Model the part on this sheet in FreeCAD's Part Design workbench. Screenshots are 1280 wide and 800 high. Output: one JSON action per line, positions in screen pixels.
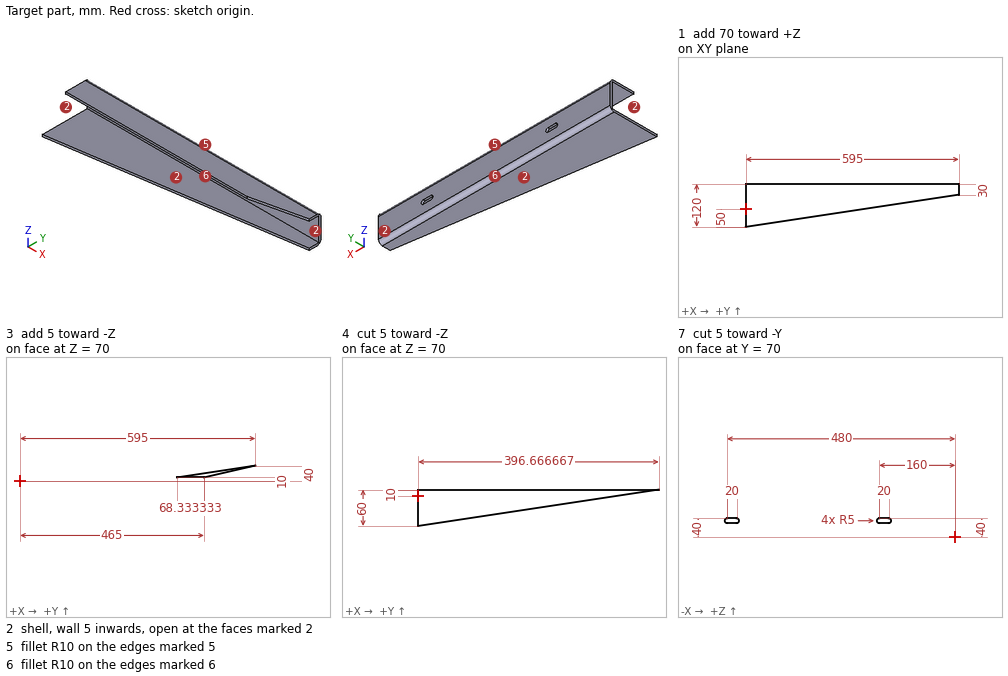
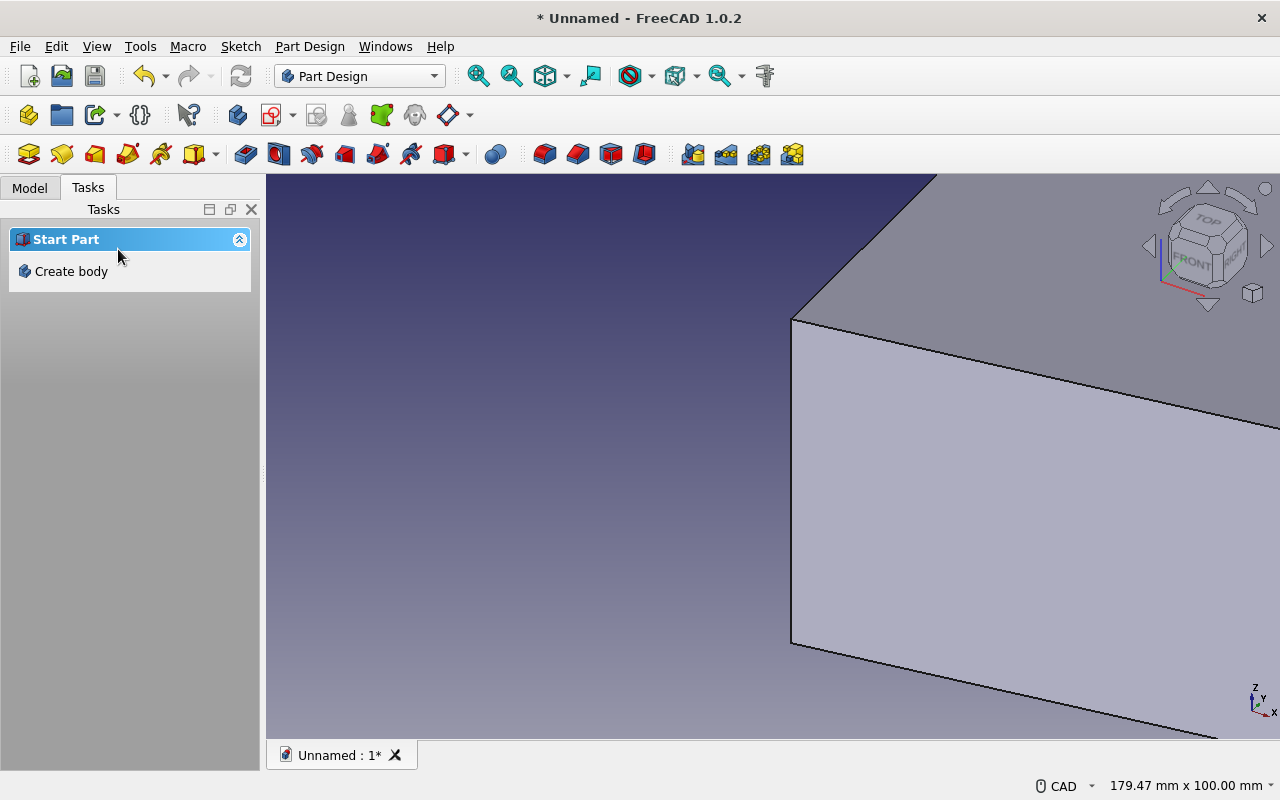
{"action": "left_click", "coordinate": [479, 76]}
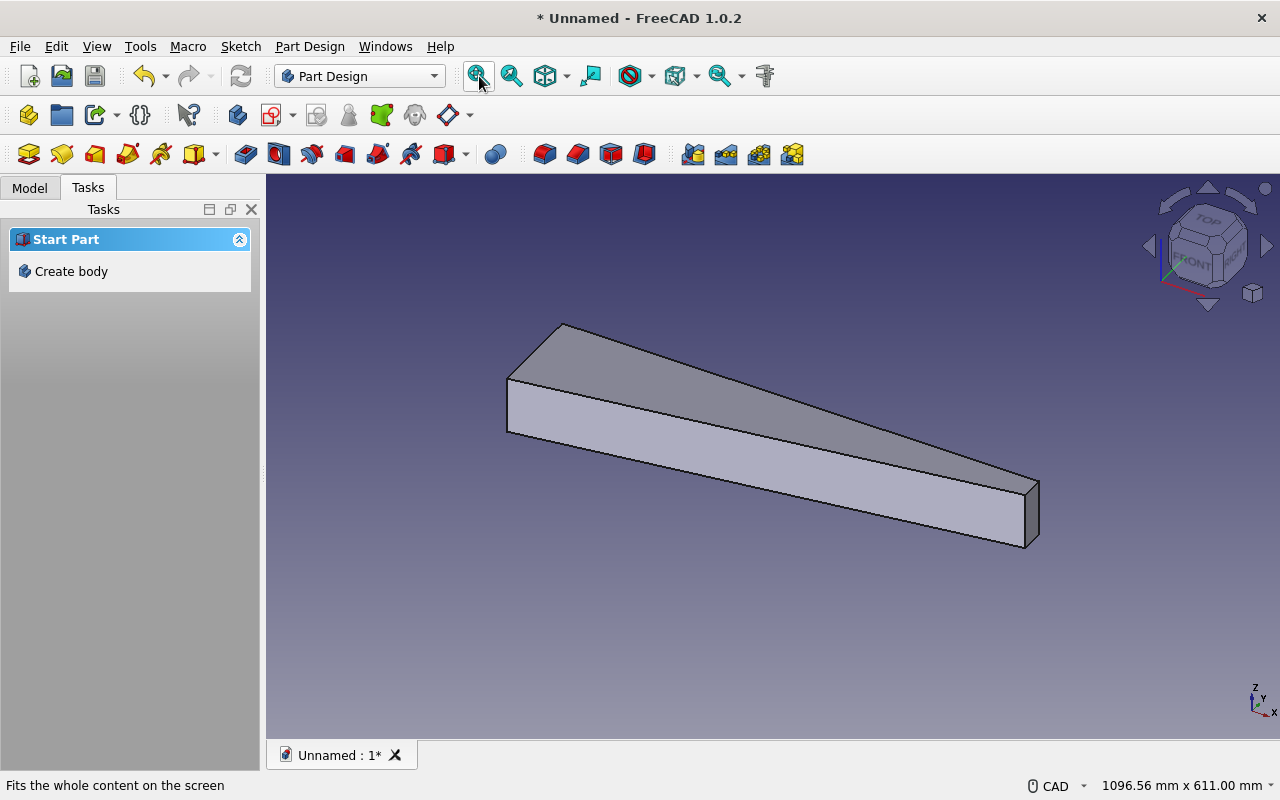
{"action": "left_click", "coordinate": [1034, 504]}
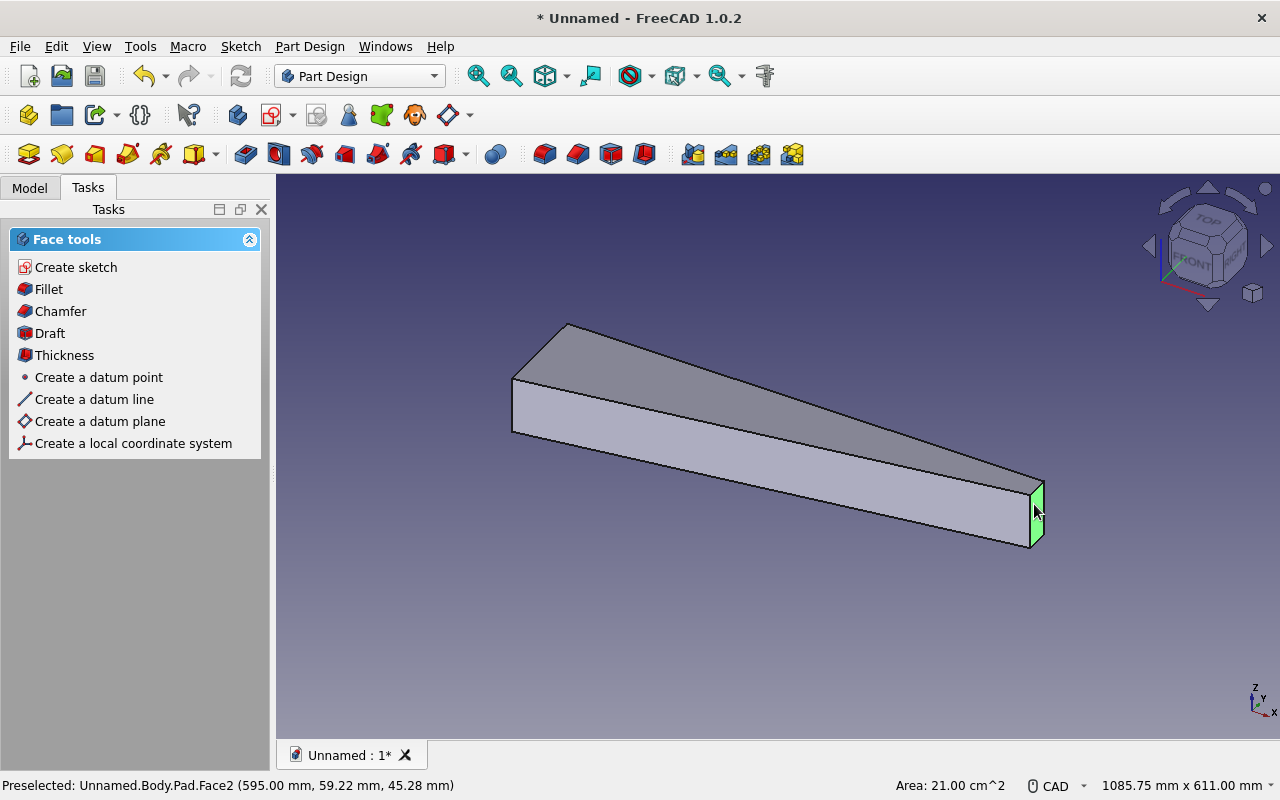
{"action": "left_click", "coordinate": [993, 512], "text": "ctrl"}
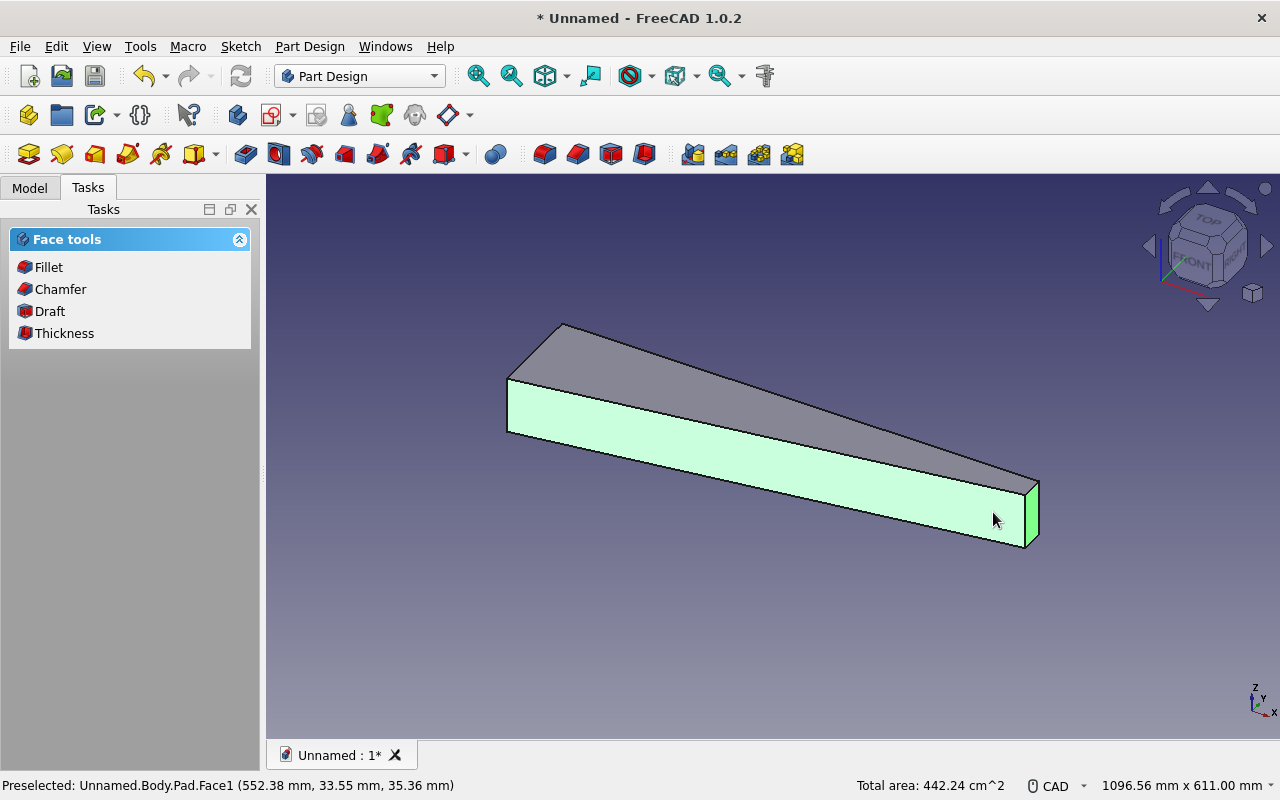
{"action": "key", "text": "0"}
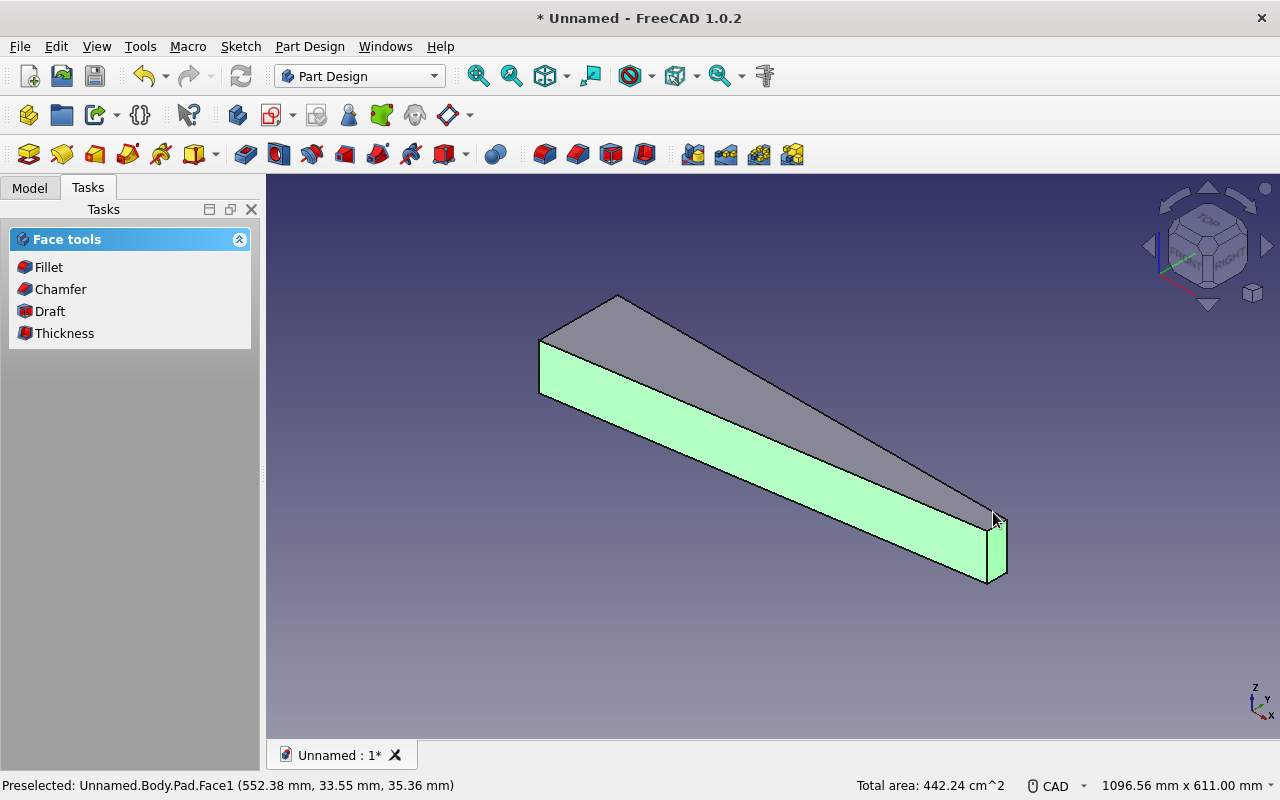
{"action": "key", "text": "2"}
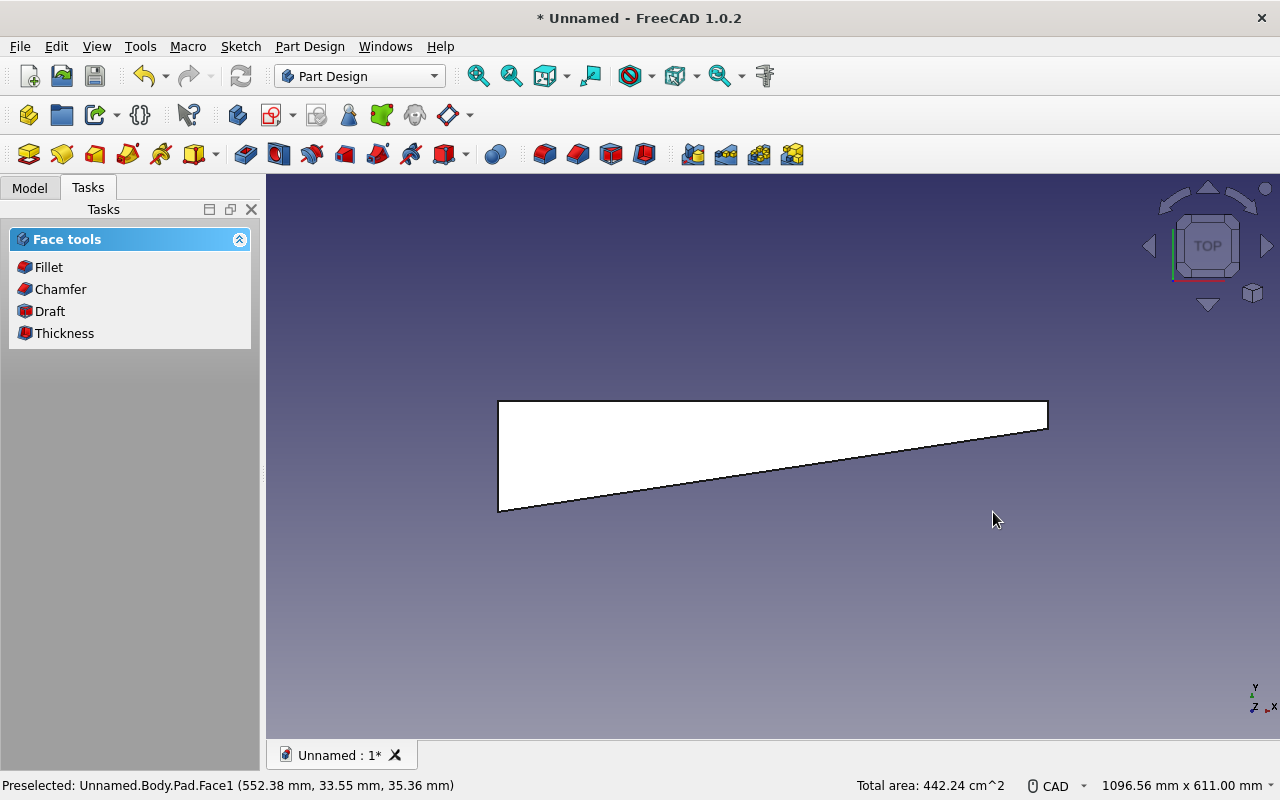
{"action": "key", "text": "1"}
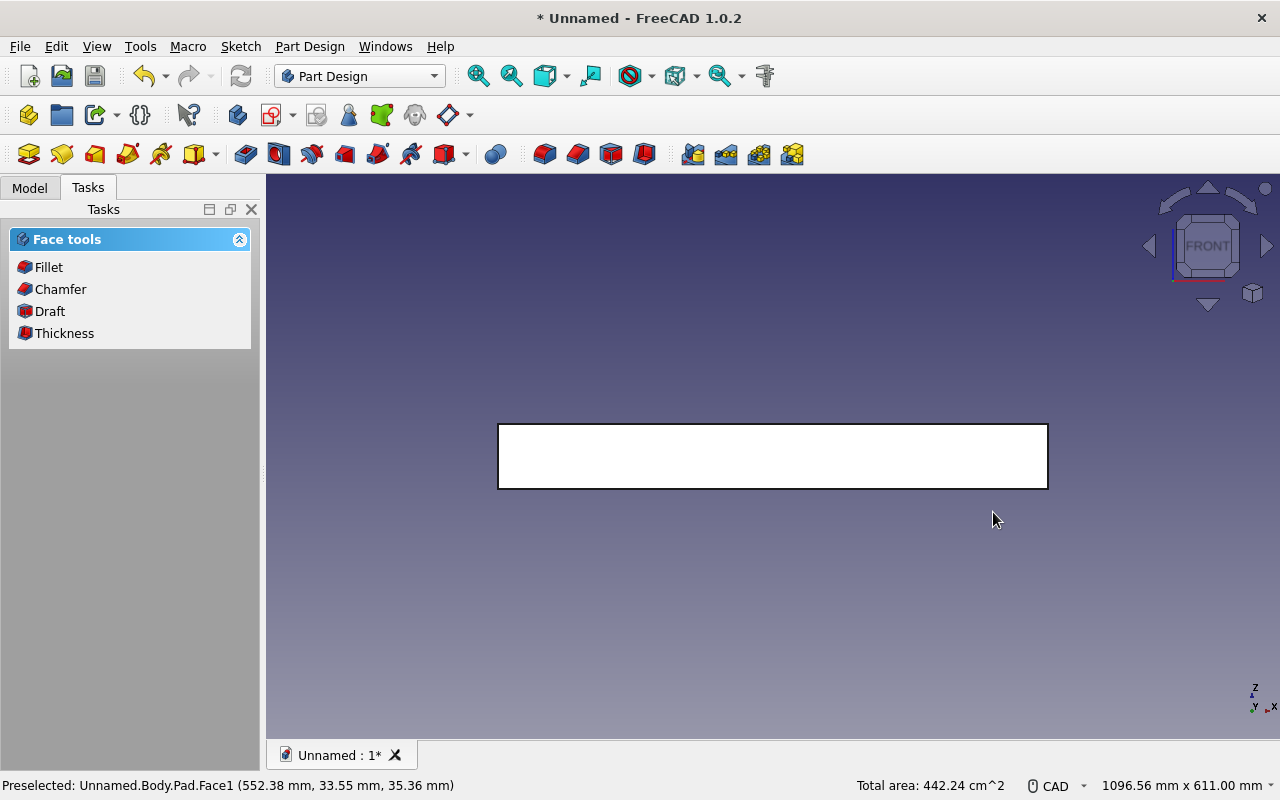
{"action": "key", "text": "3"}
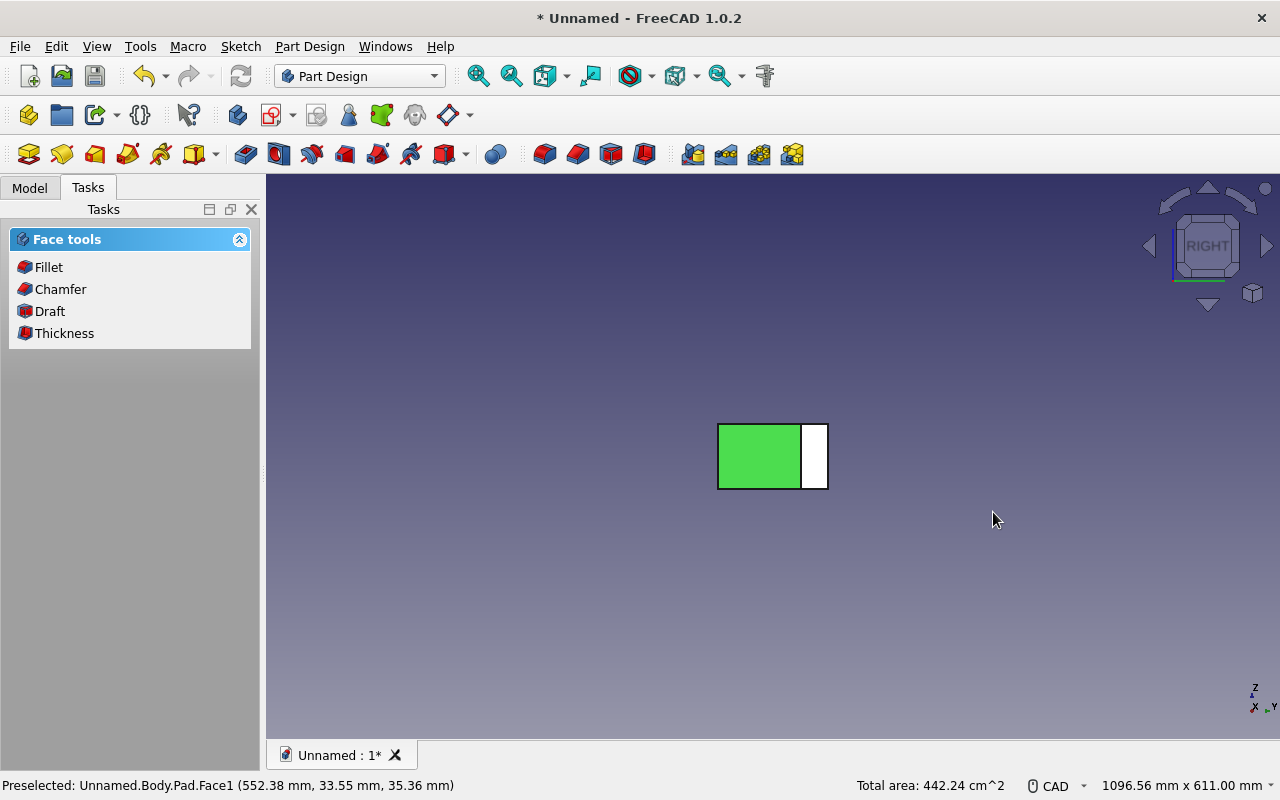
{"action": "left_click", "coordinate": [479, 76]}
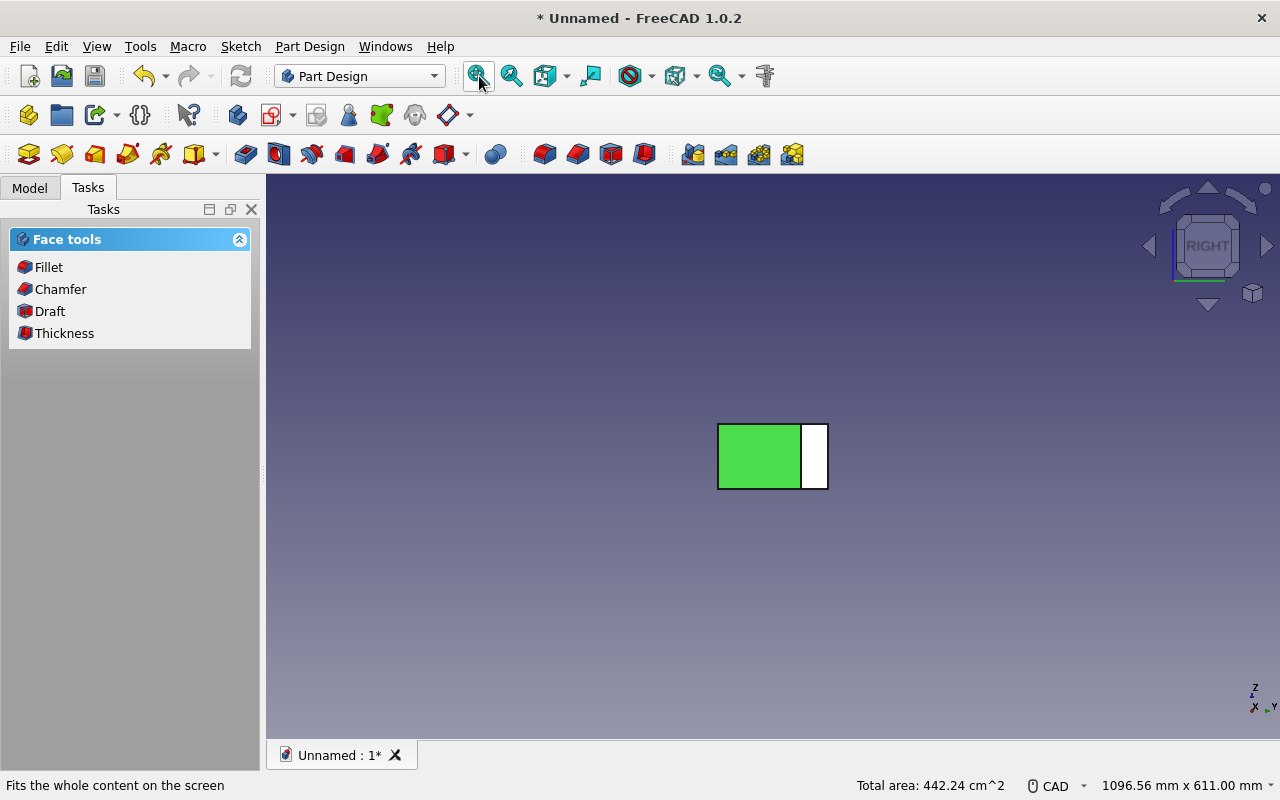
{"action": "key", "text": "5"}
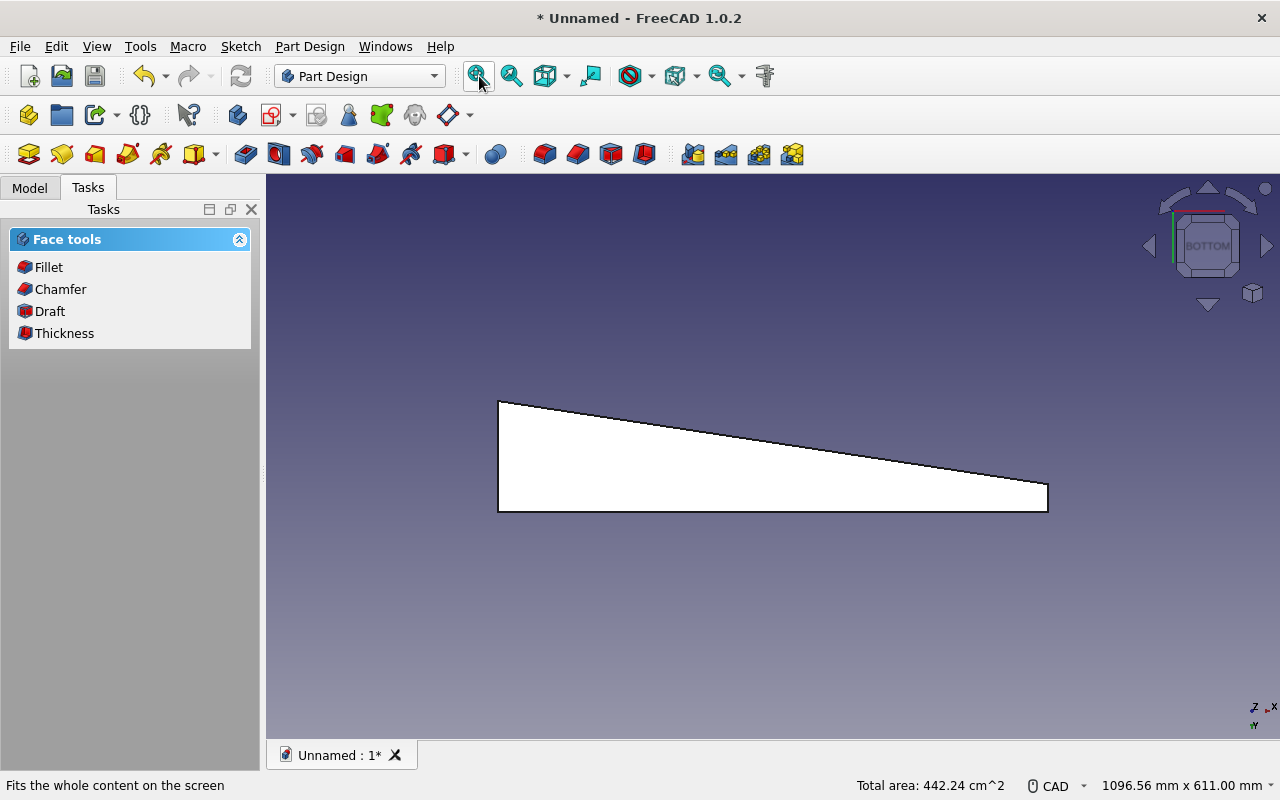
{"action": "key", "text": "4"}